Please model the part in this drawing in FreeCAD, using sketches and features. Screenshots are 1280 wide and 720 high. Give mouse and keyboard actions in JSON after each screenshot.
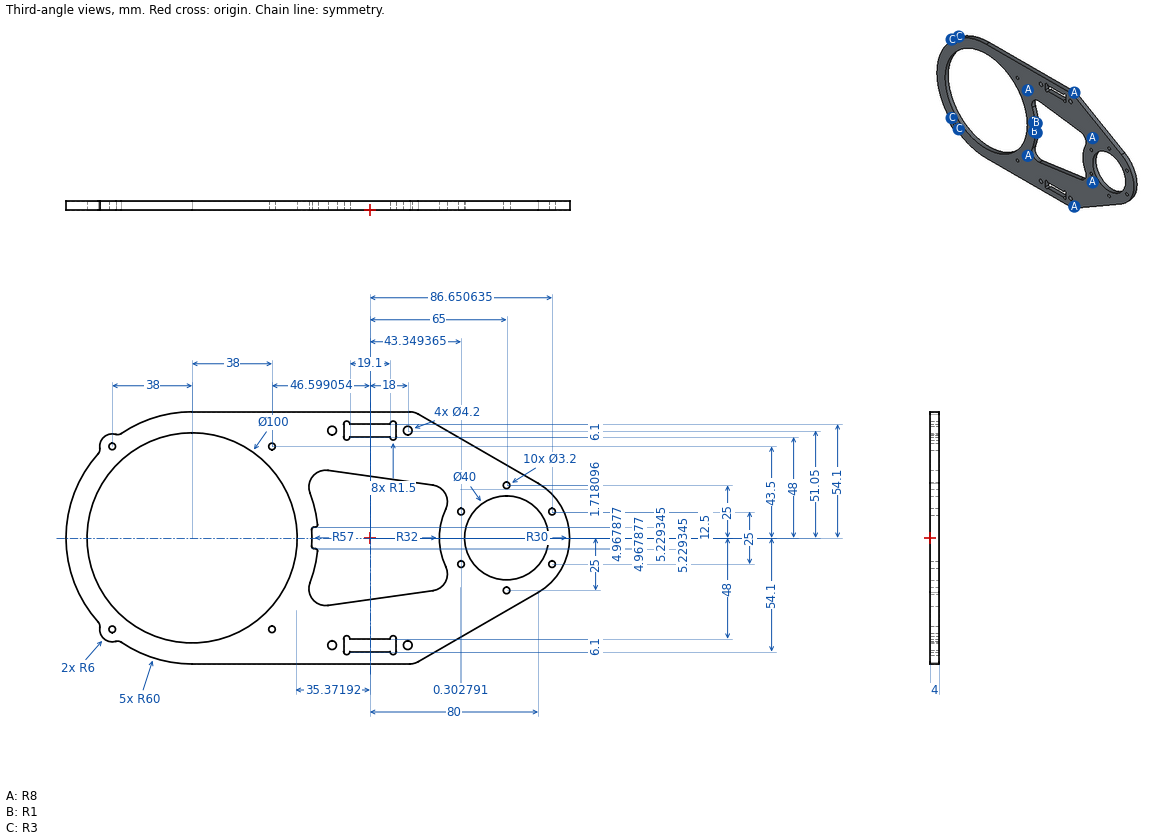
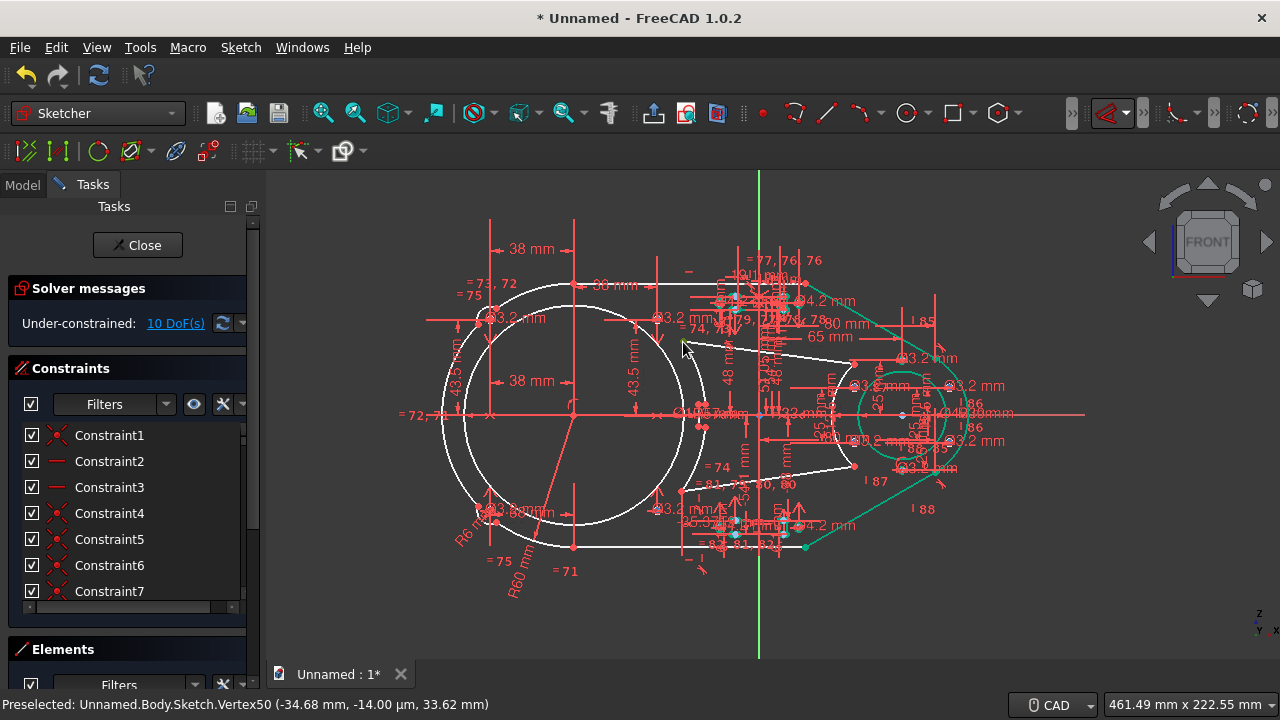
{"action": "left_click", "coordinate": [1128, 114]}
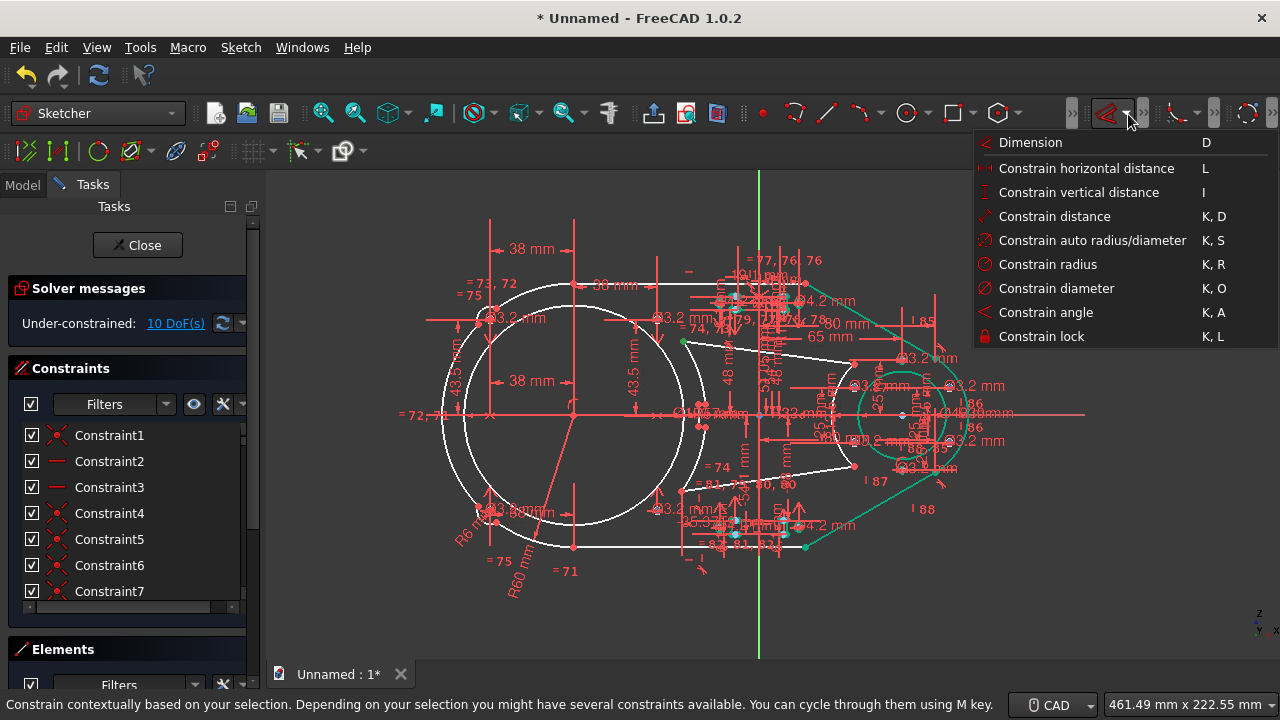
{"action": "left_click", "coordinate": [1126, 168]}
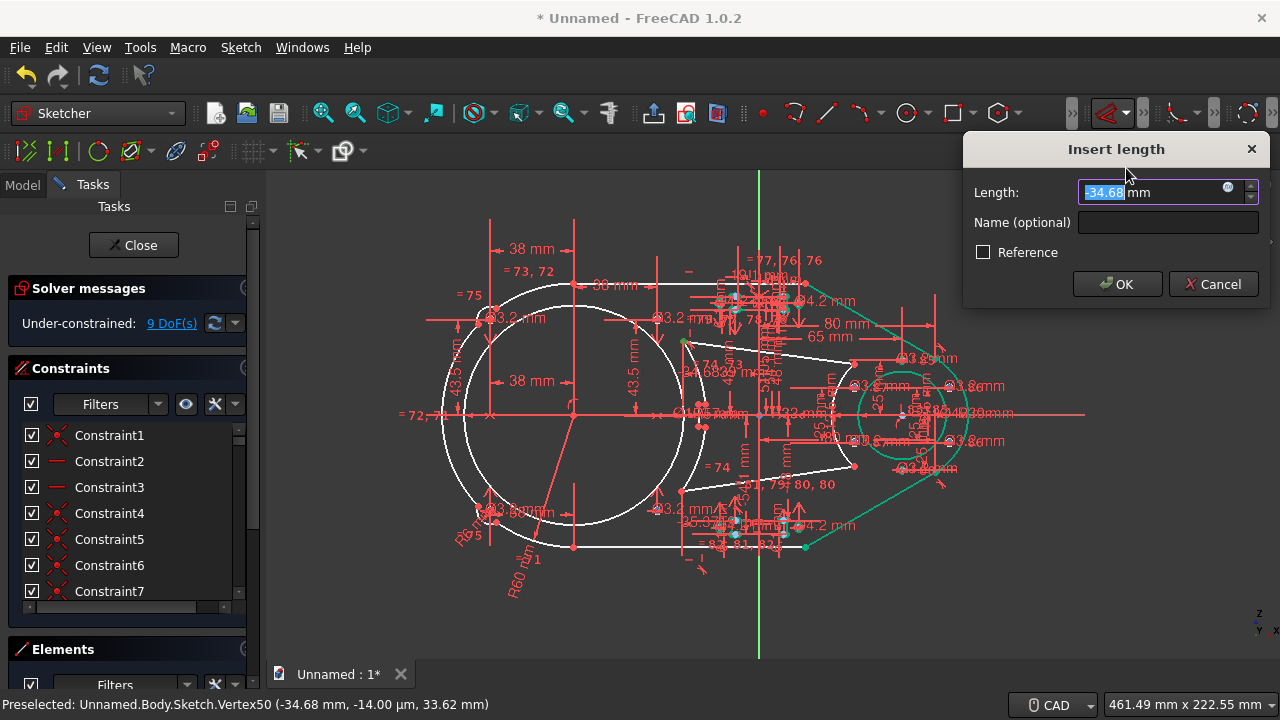
{"action": "type", "text": "-35.37192"}
{"action": "key", "text": "Return"}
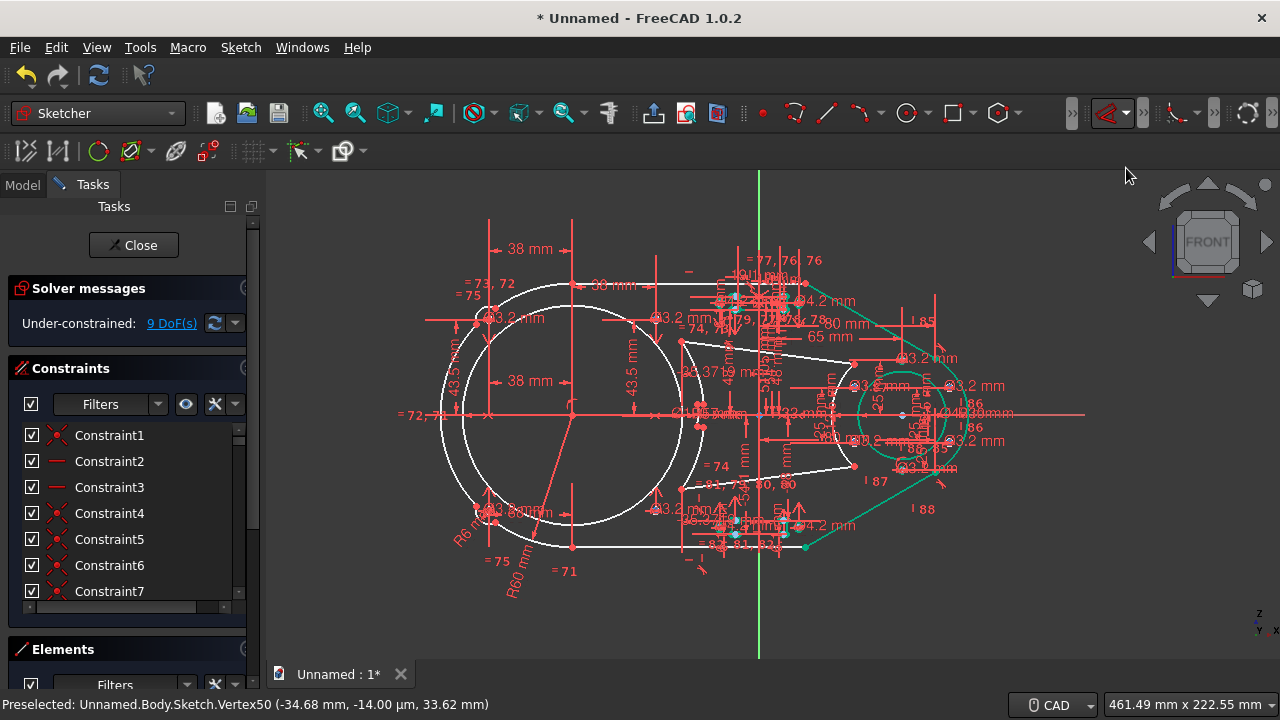
{"action": "scroll", "coordinate": [704, 404], "scroll_direction": "up", "scroll_amount": 7}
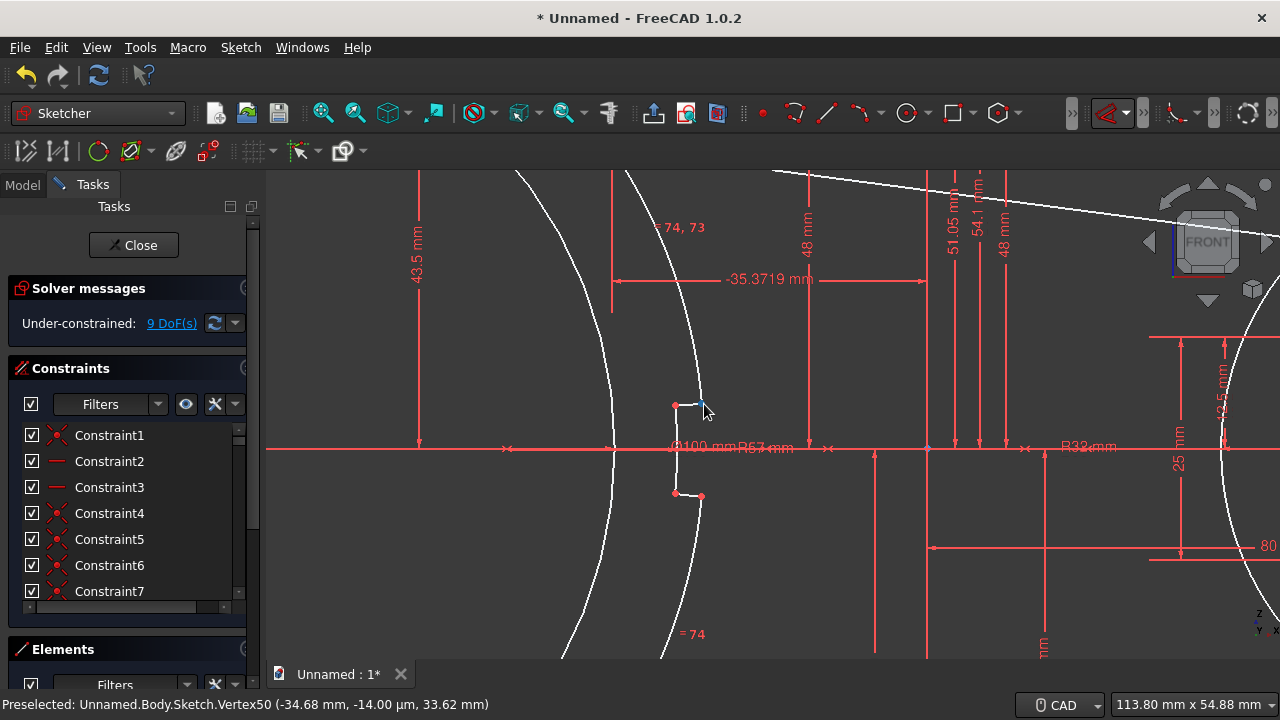
{"action": "left_click", "coordinate": [702, 404]}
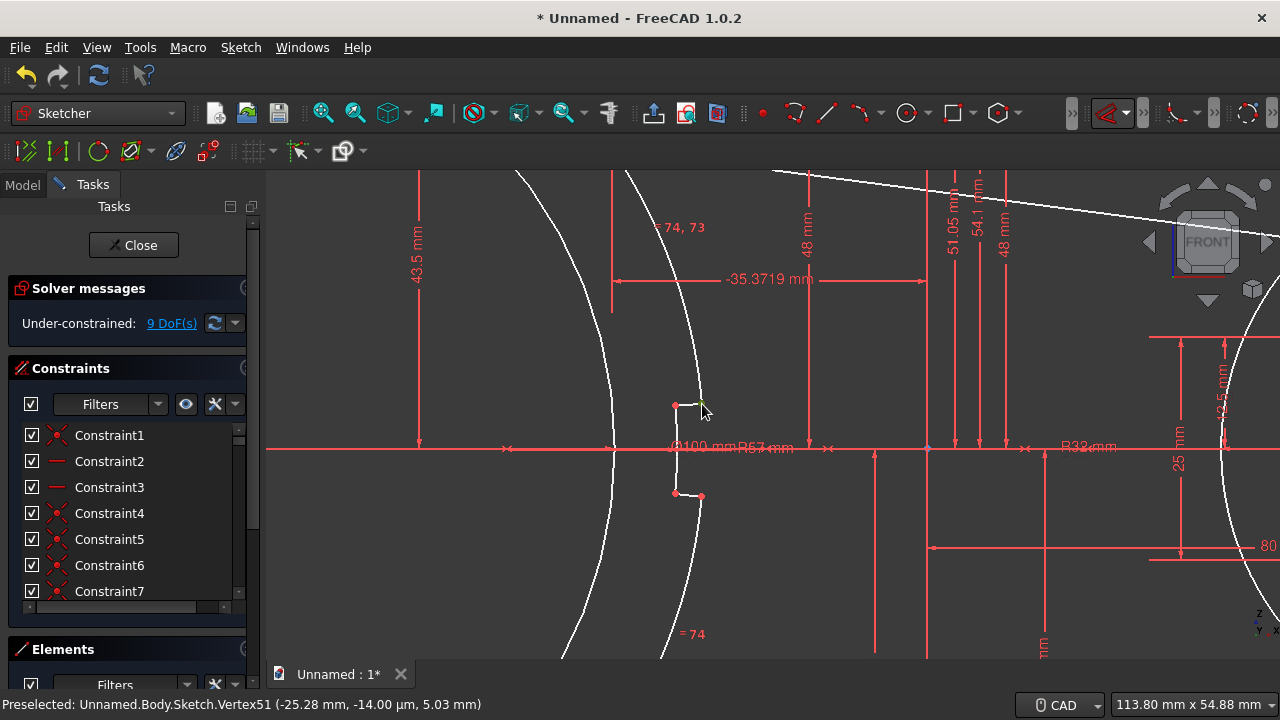
{"action": "left_click", "coordinate": [1128, 114]}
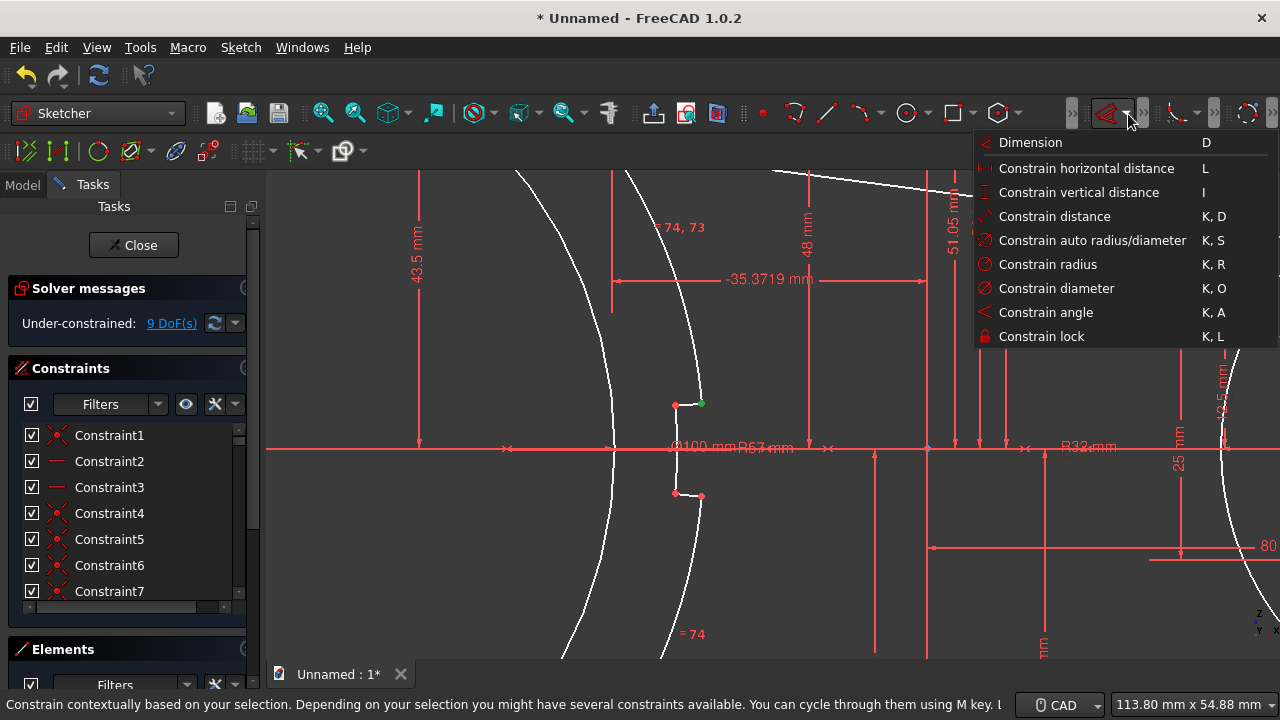
{"action": "left_click", "coordinate": [1126, 192]}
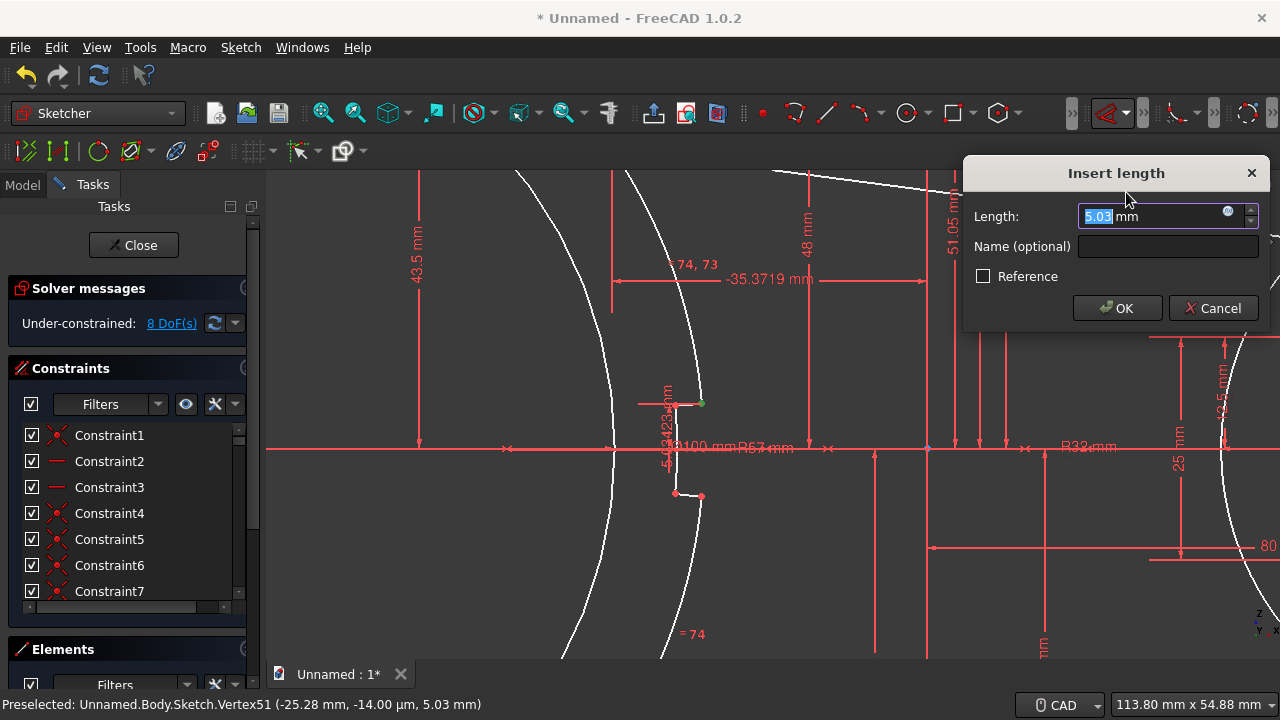
{"action": "type", "text": "5.229345"}
{"action": "key", "text": "Return"}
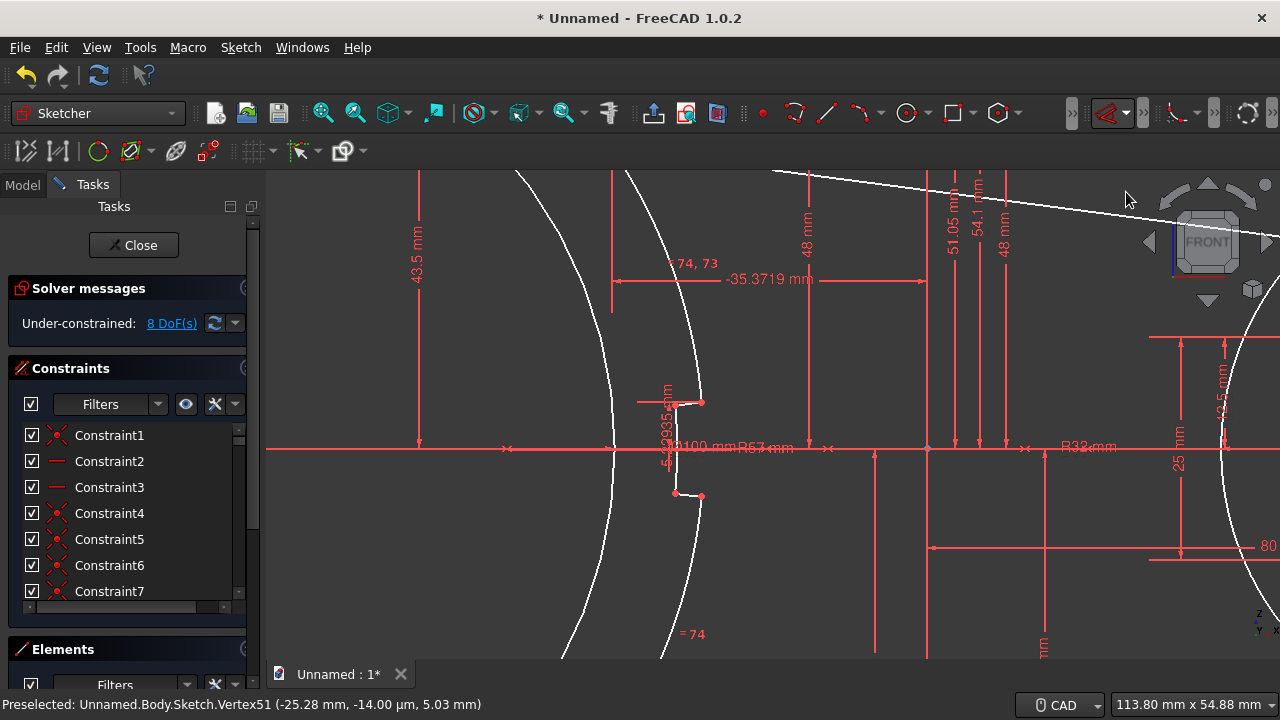
{"action": "left_click", "coordinate": [675, 406]}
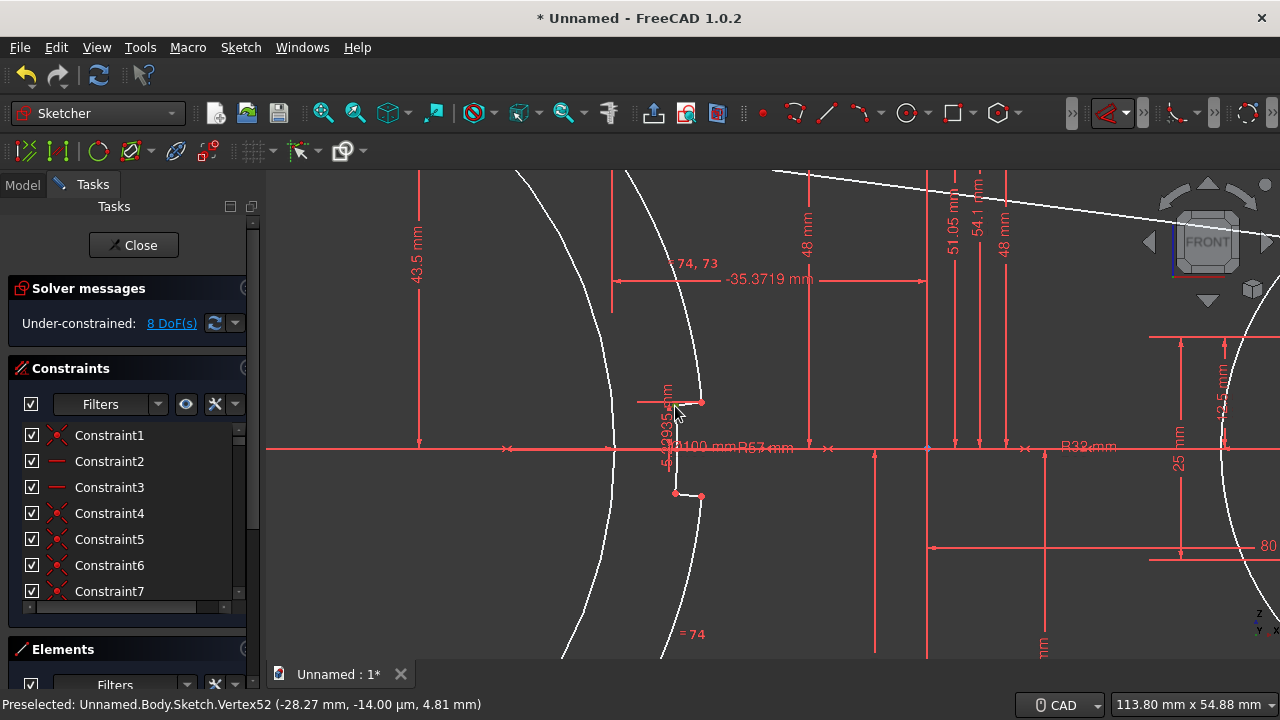
{"action": "key", "text": "i"}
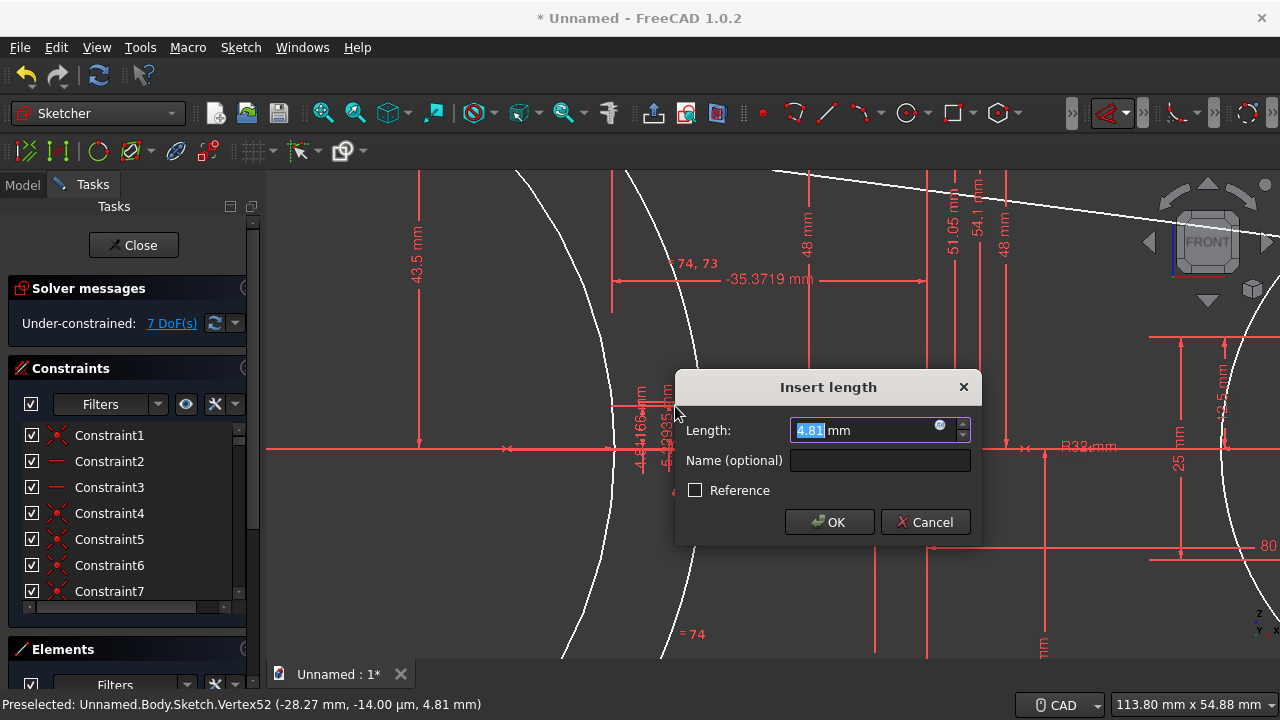
{"action": "type", "text": "4.967877"}
{"action": "key", "text": "Return"}